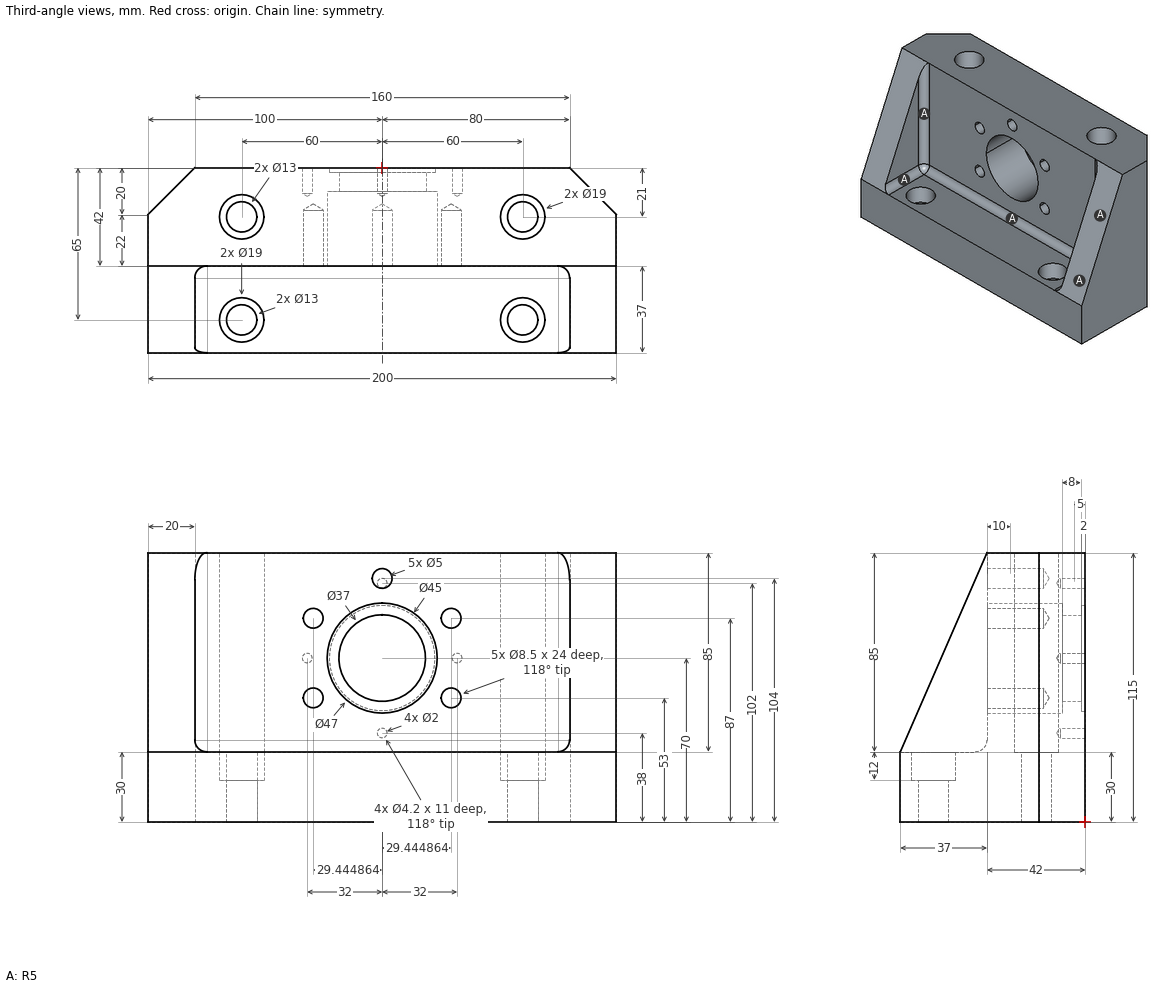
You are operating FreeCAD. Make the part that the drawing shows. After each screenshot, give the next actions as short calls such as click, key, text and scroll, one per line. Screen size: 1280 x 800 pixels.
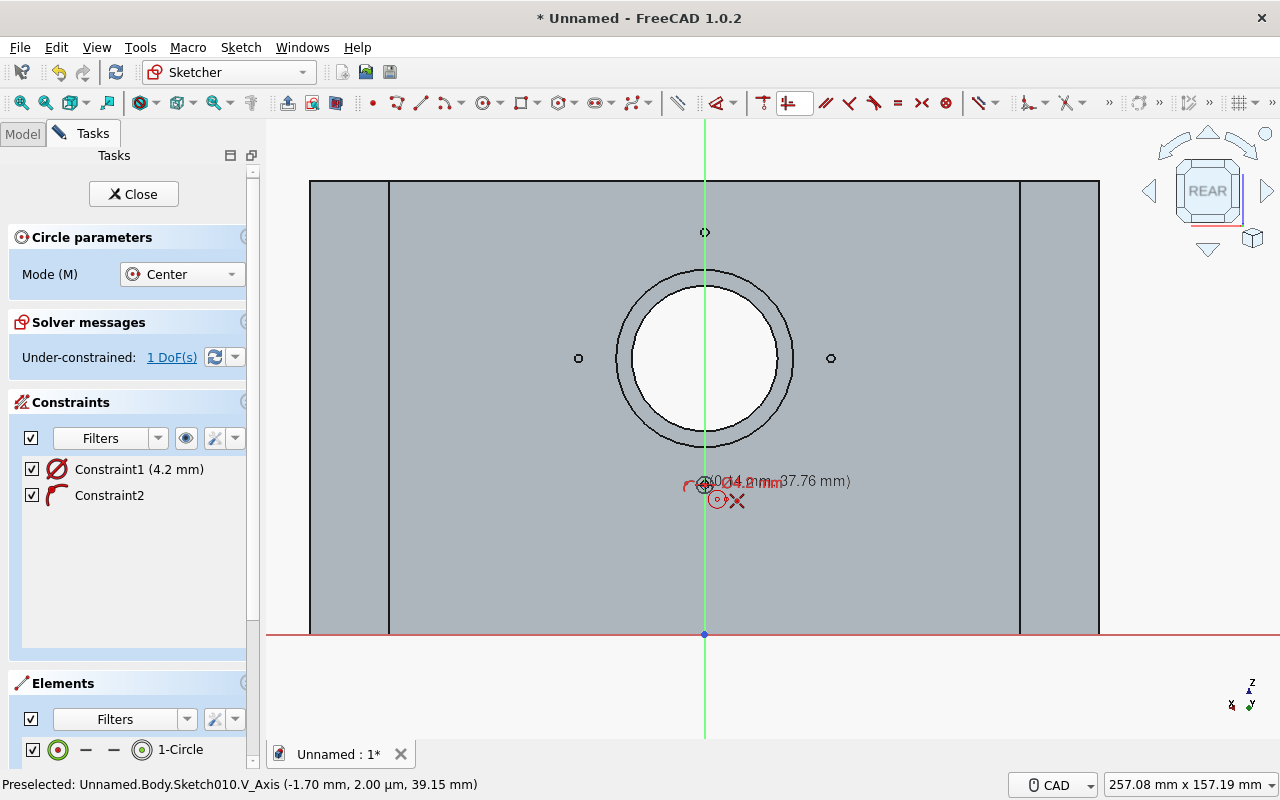
scroll(579, 359, up, 6)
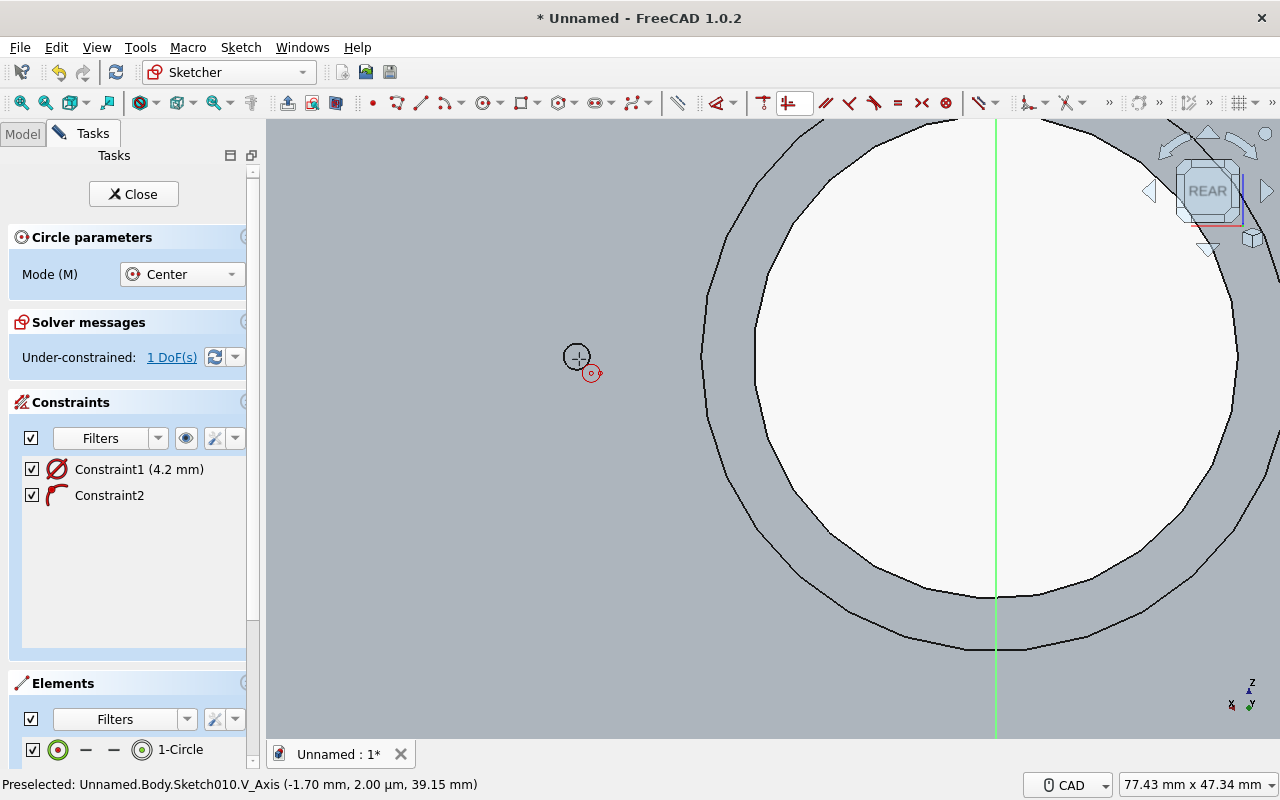
click(577, 357)
move(596, 337)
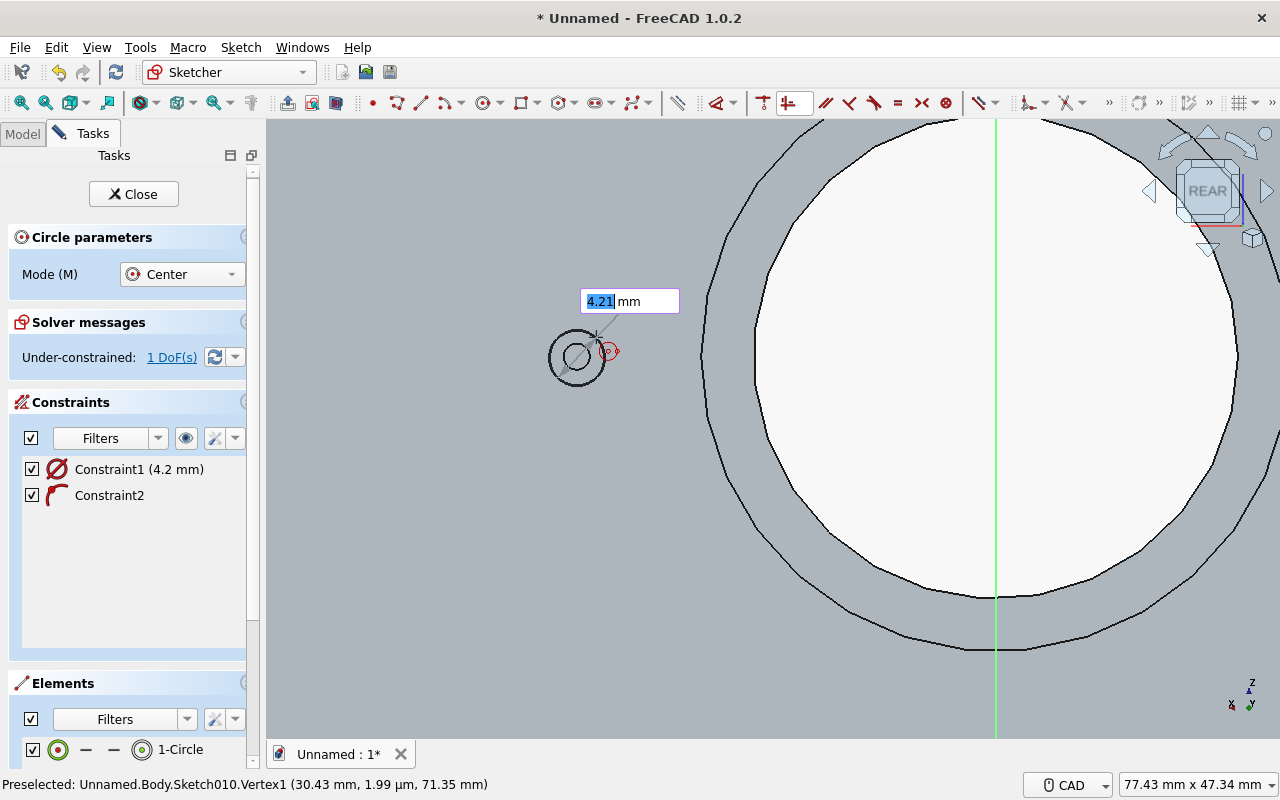
text(4.2)
key(Return)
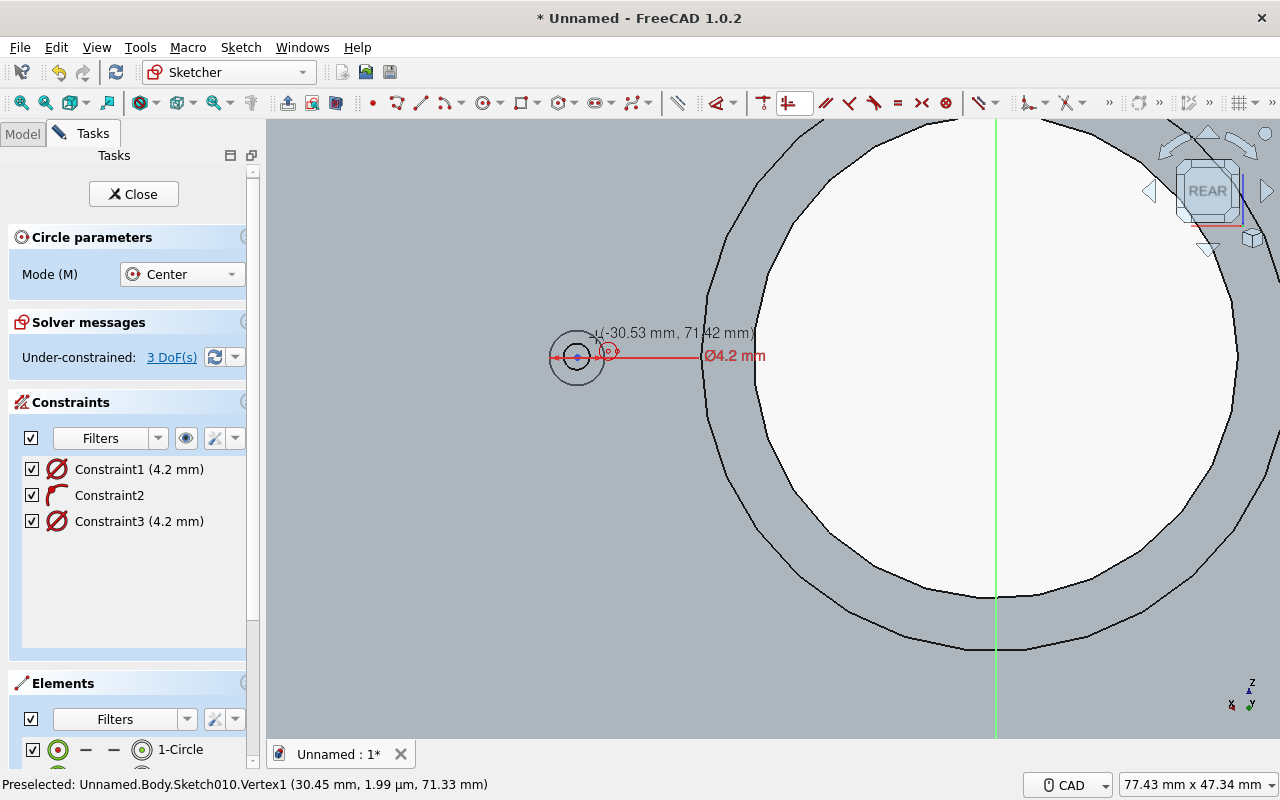
scroll(579, 359, down, 6)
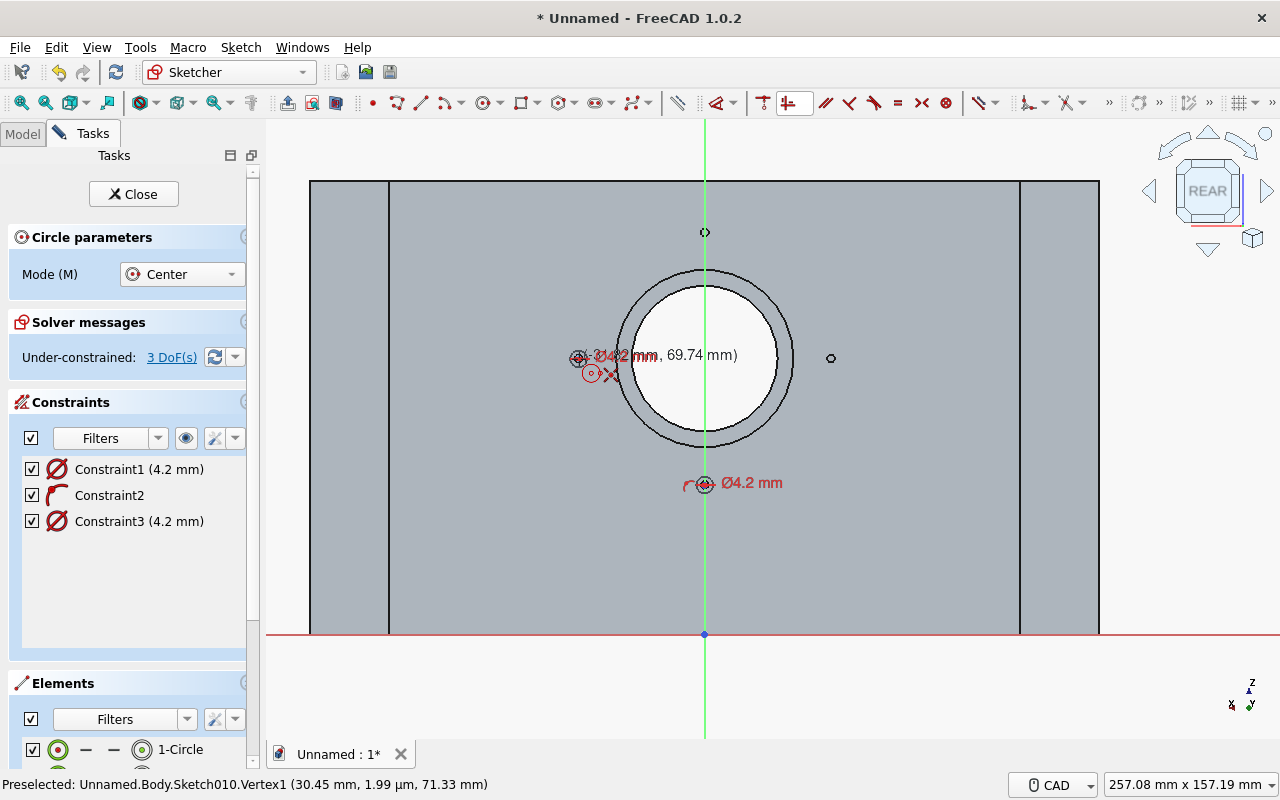
scroll(705, 232, up, 6)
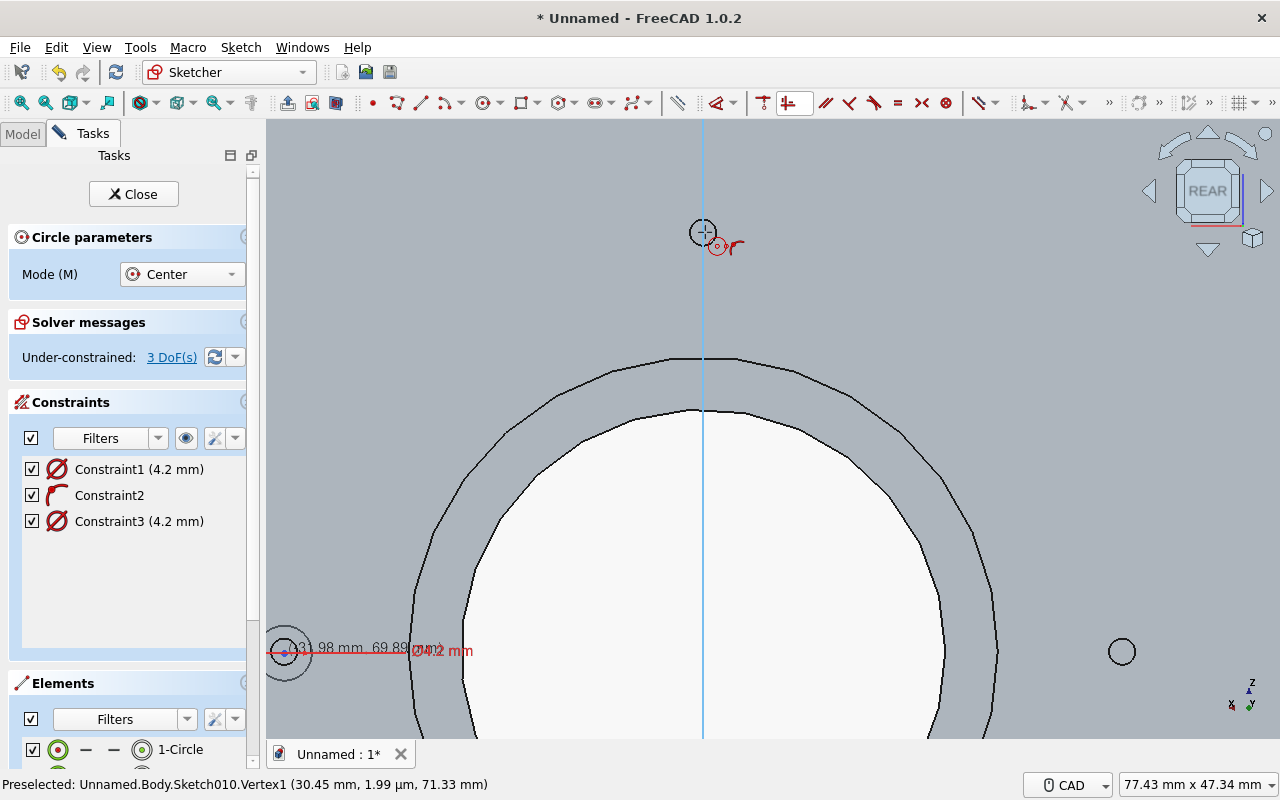
click(703, 233)
move(723, 213)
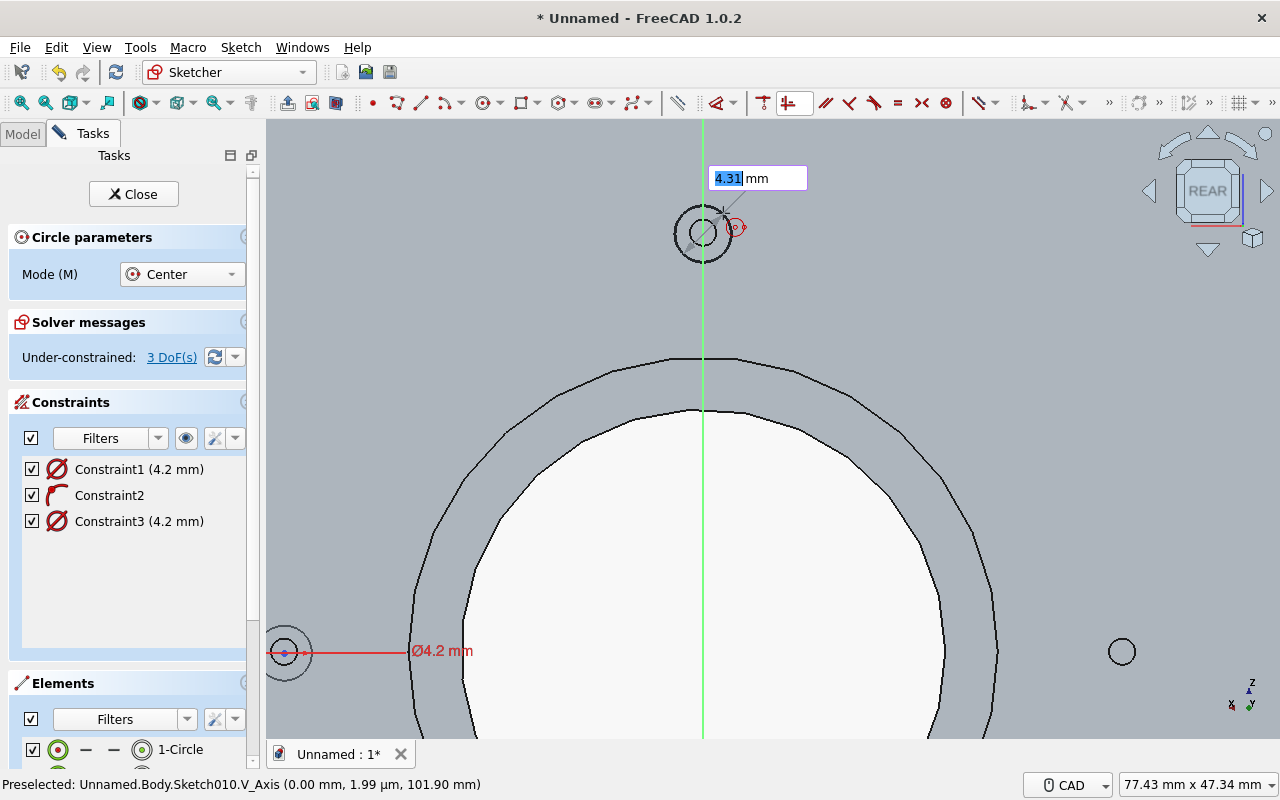
text(4.2)
key(Return)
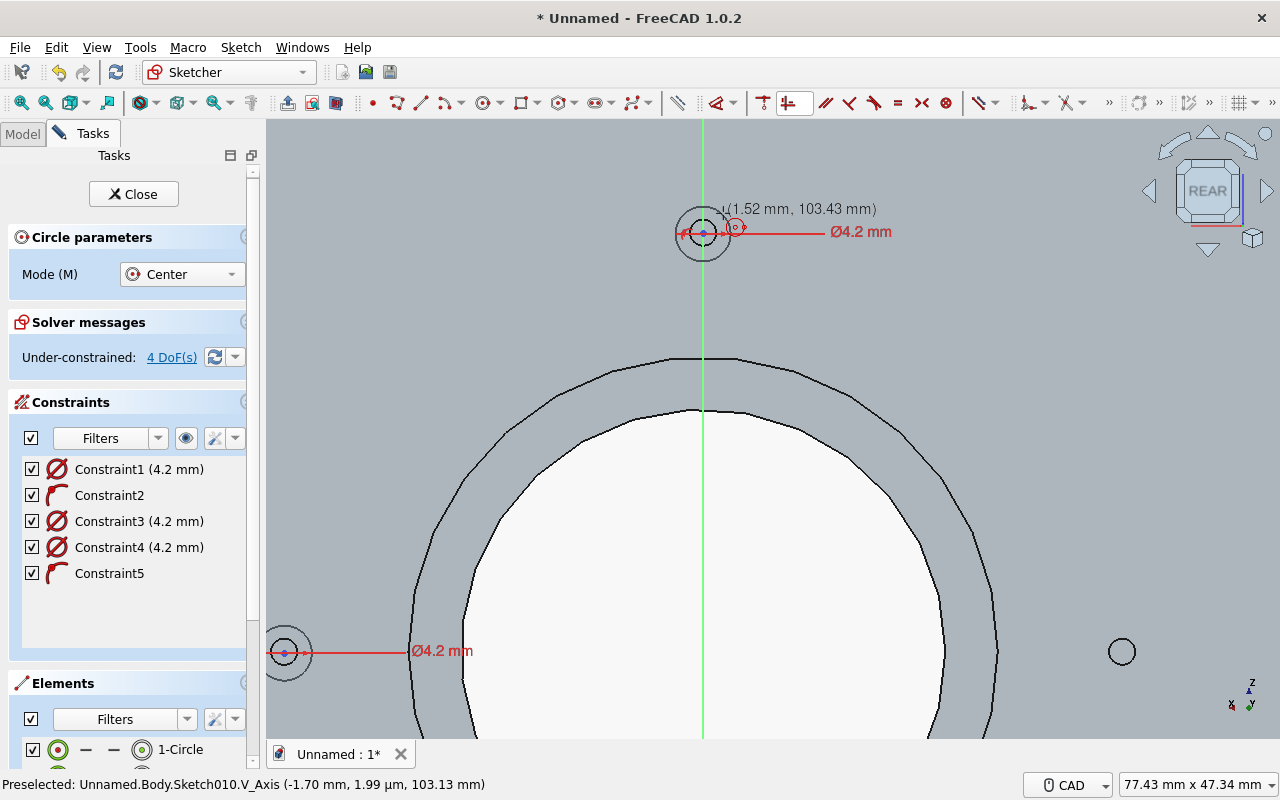
scroll(705, 232, down, 6)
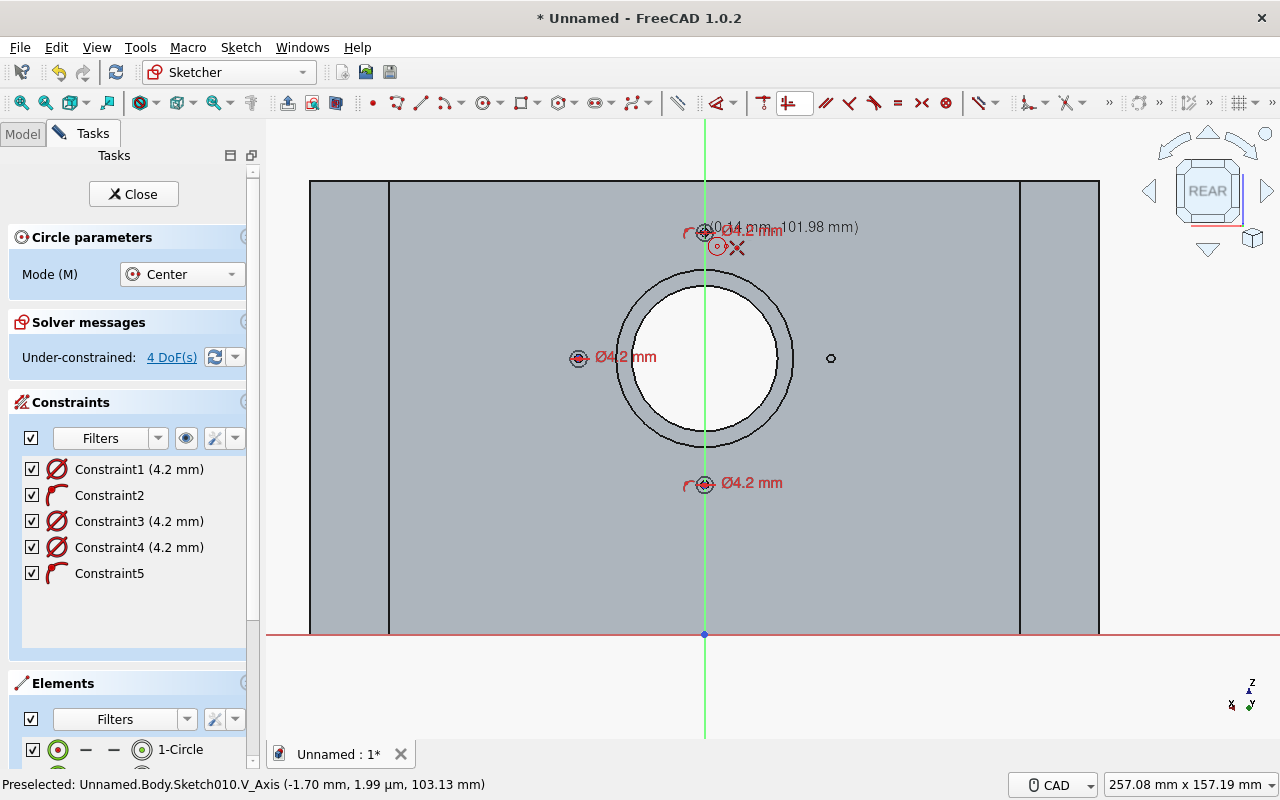
scroll(831, 359, up, 6)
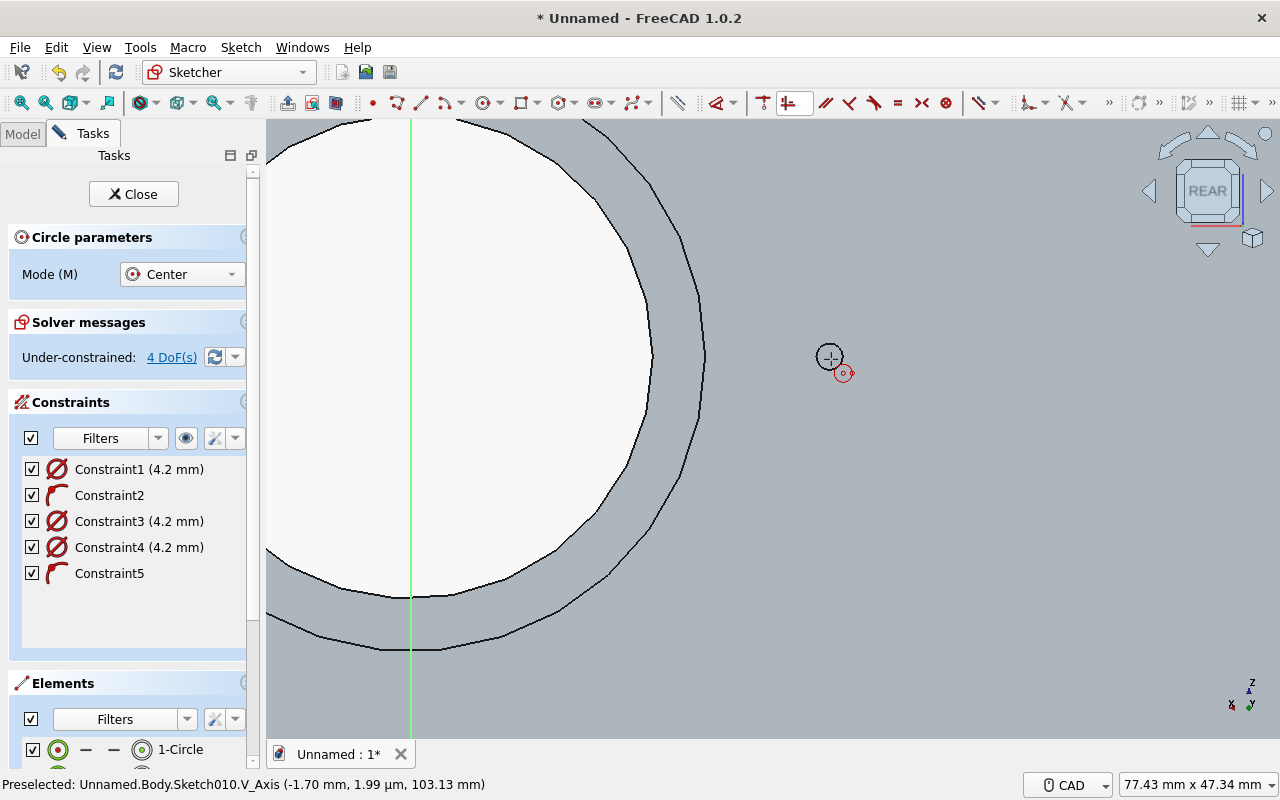
click(830, 357)
move(849, 337)